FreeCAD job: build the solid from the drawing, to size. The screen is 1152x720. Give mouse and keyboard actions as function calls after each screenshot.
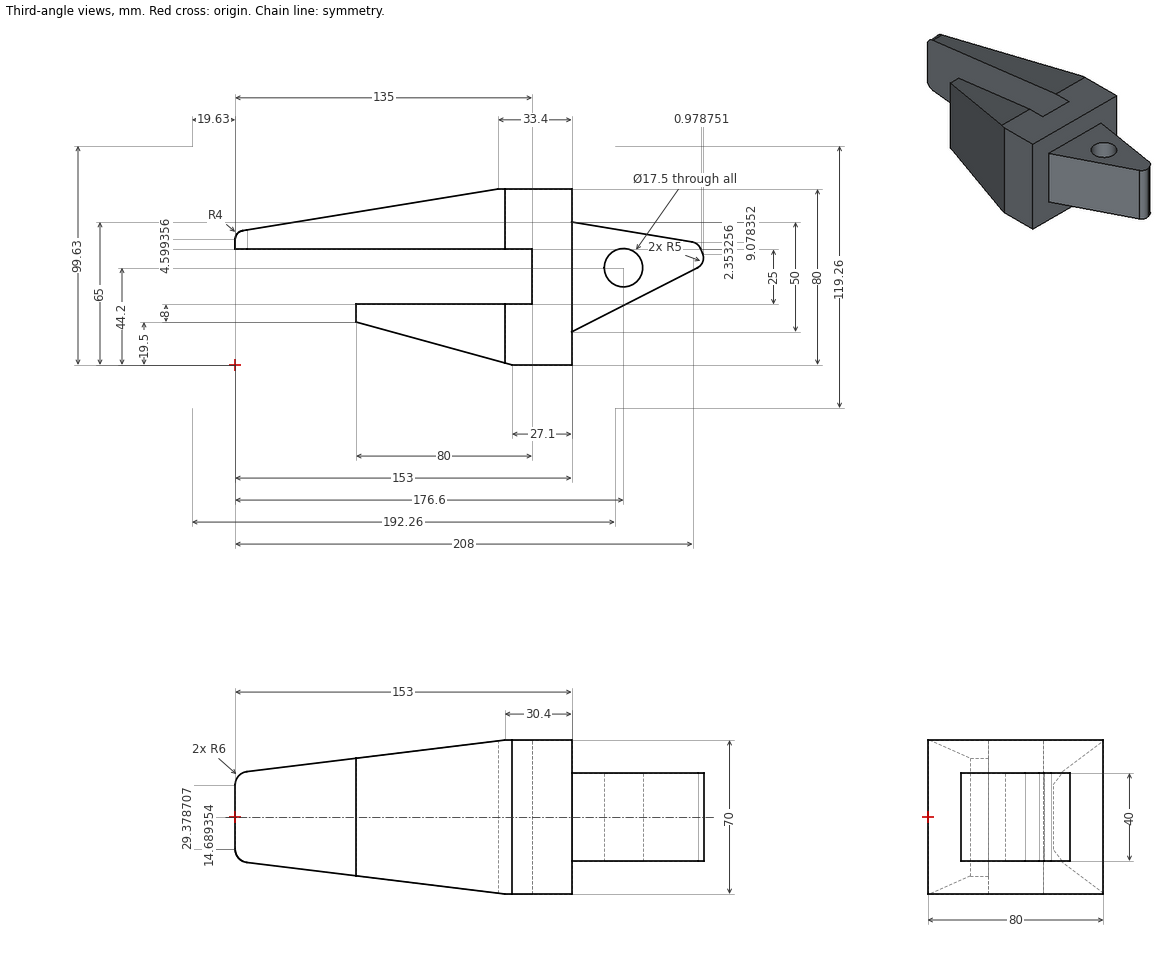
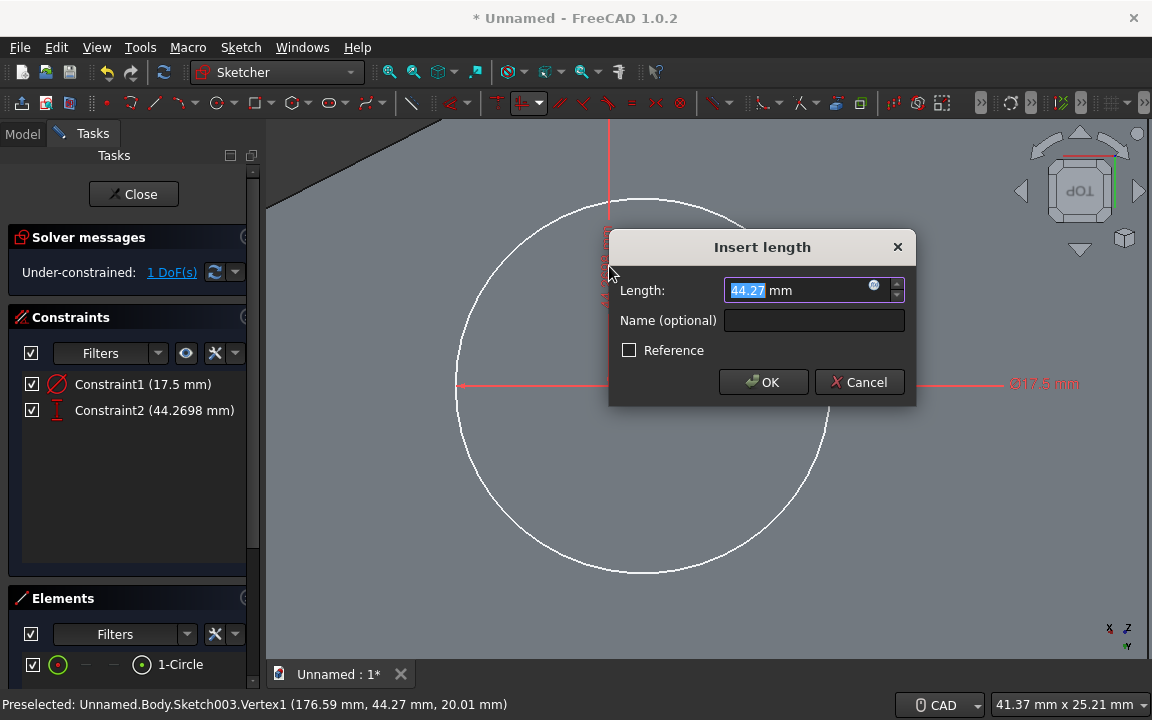
text(44.2)
key(Return)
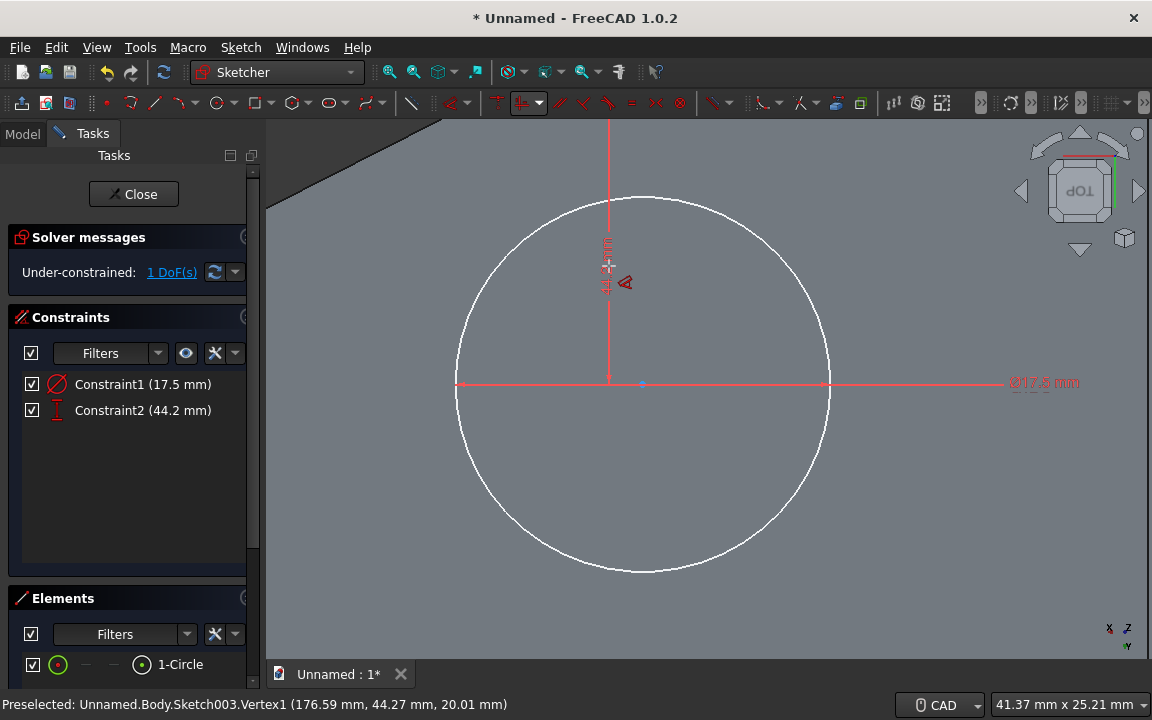
click(643, 385)
click(736, 419)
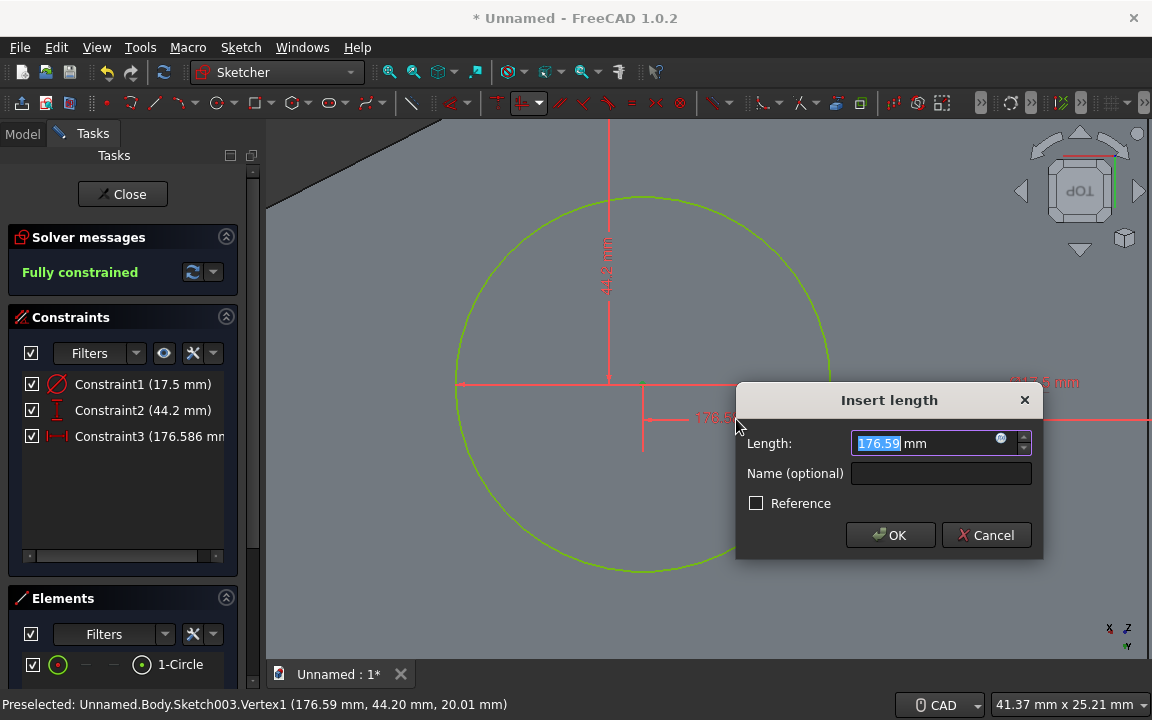
text(176.6)
key(Return)
key(Escape)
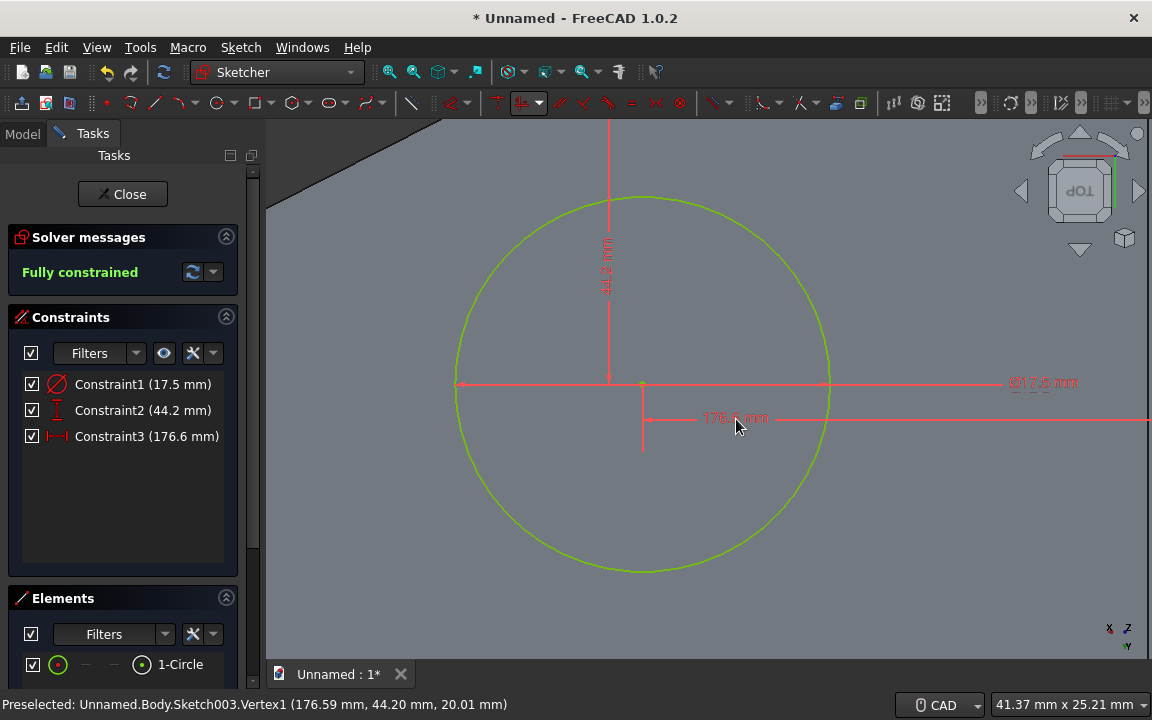
click(123, 194)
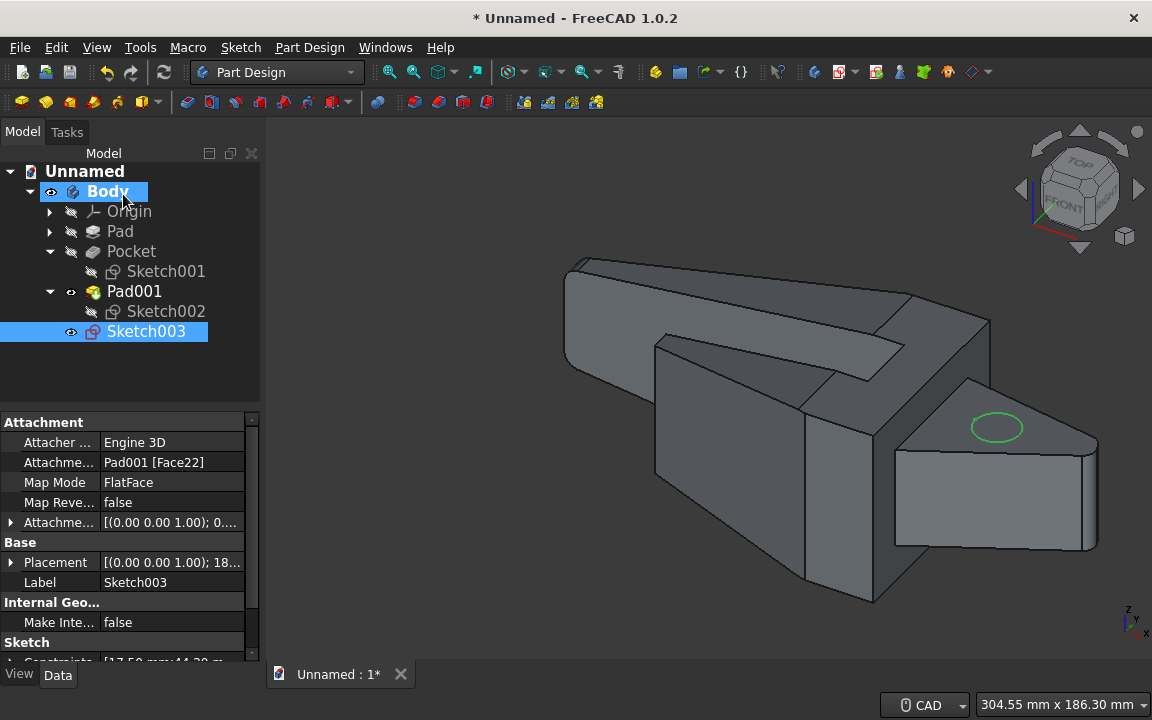
click(212, 102)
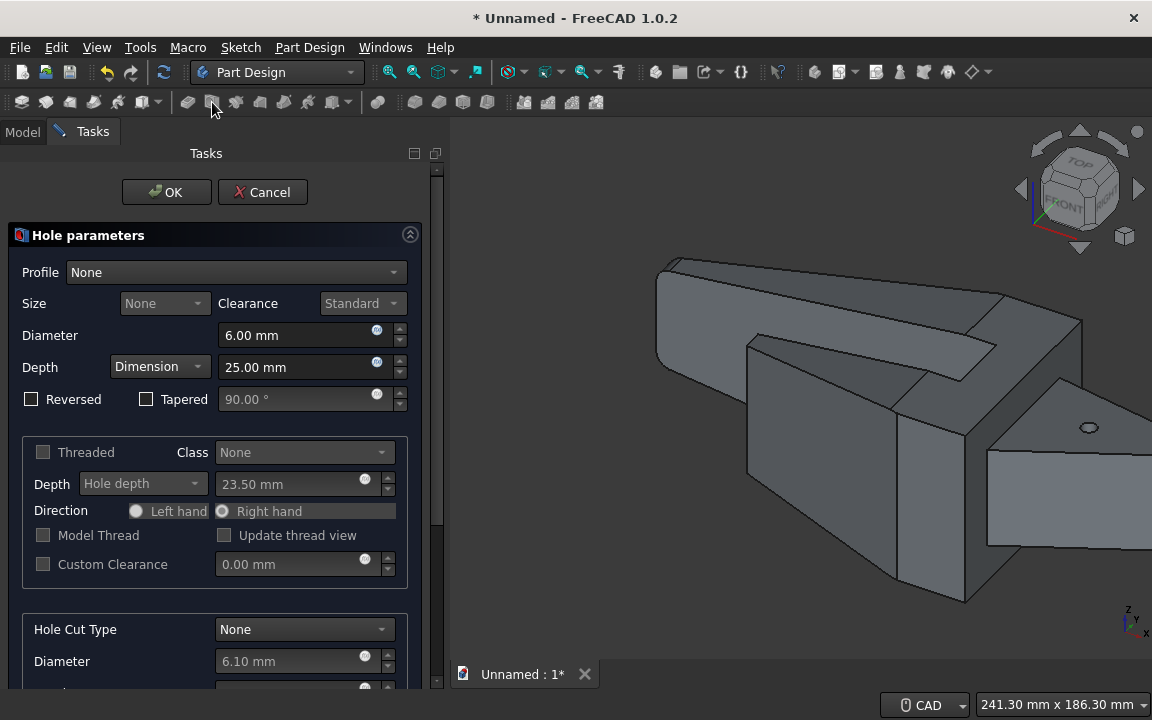
triple_click(305, 335)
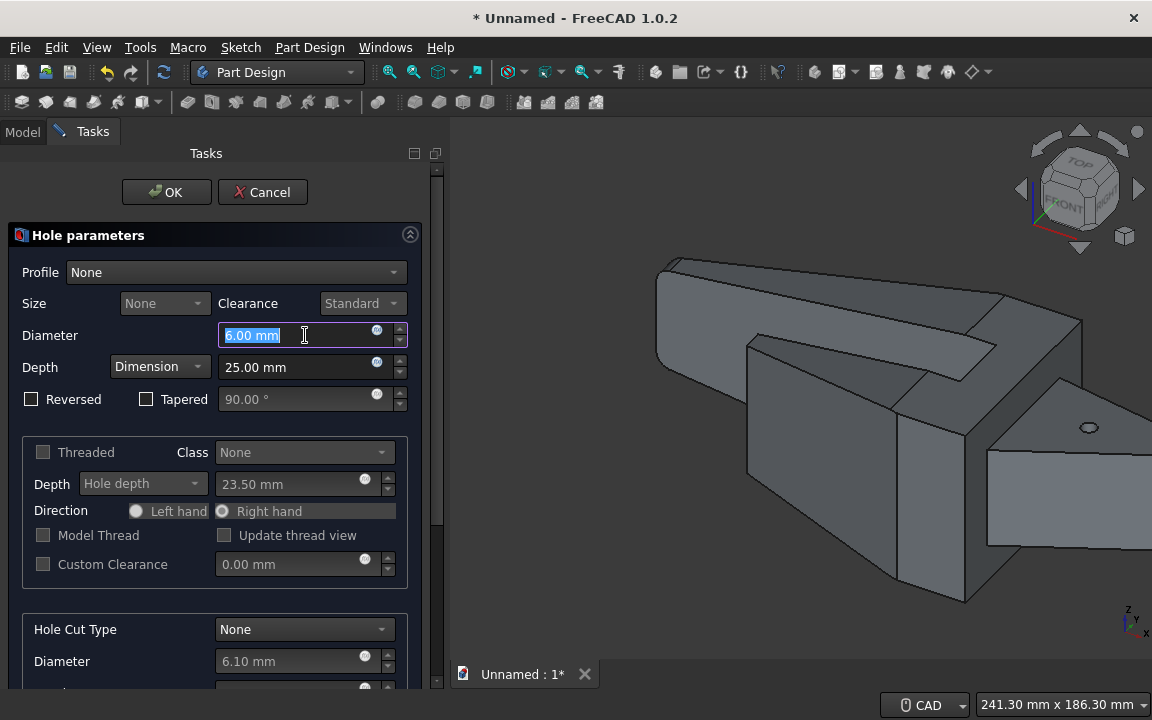
text(17.5)
key(Tab)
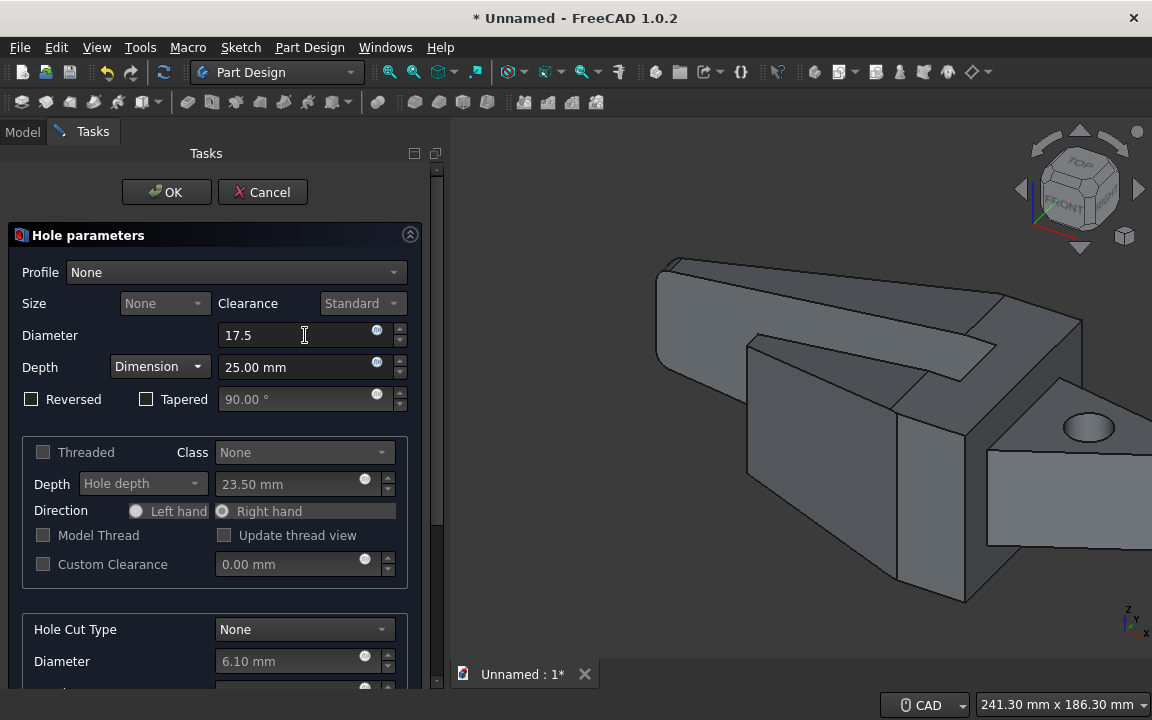
click(161, 366)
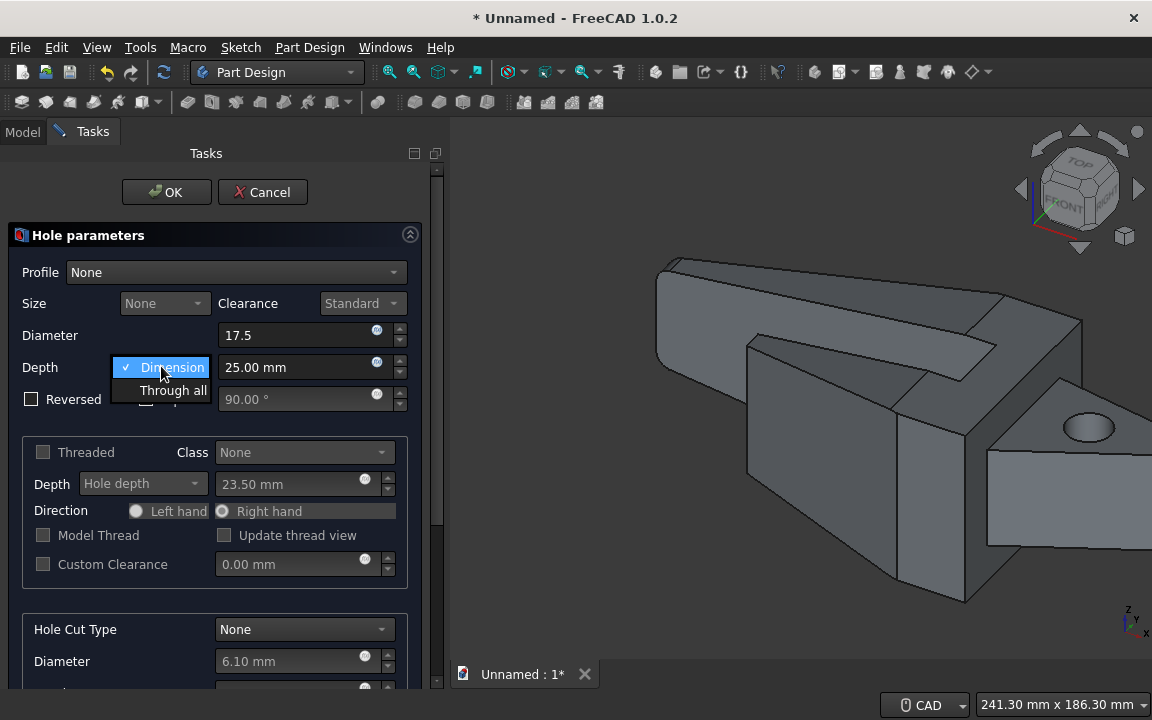
click(160, 390)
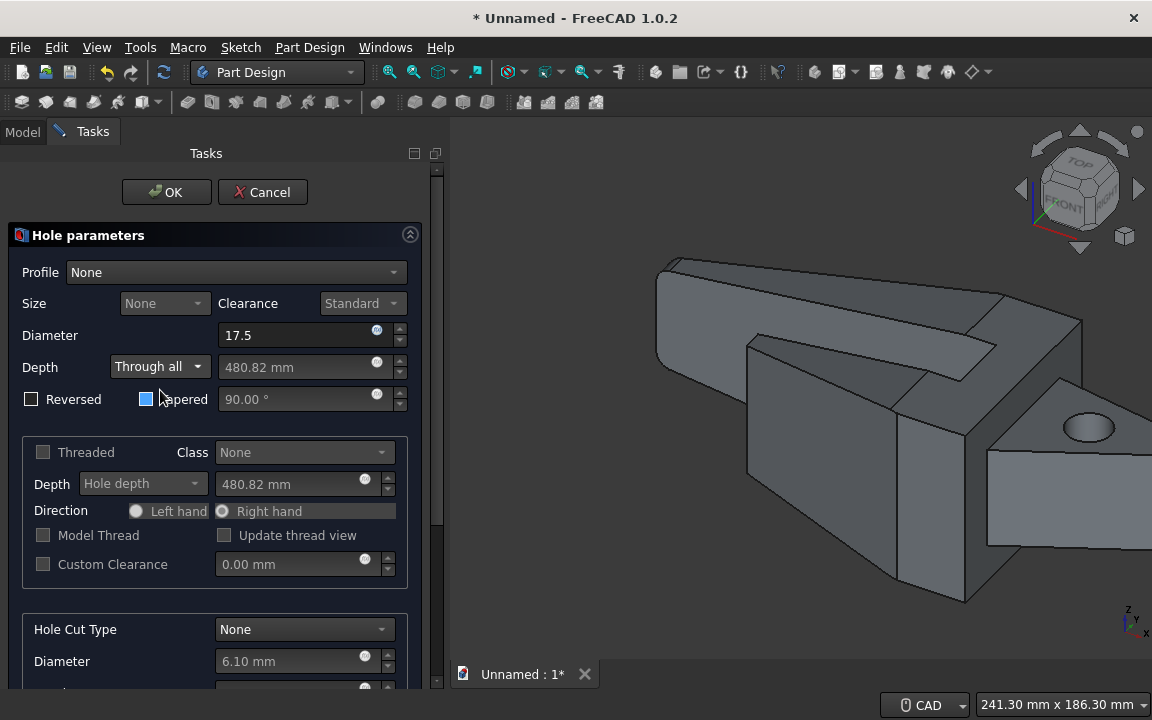
click(167, 192)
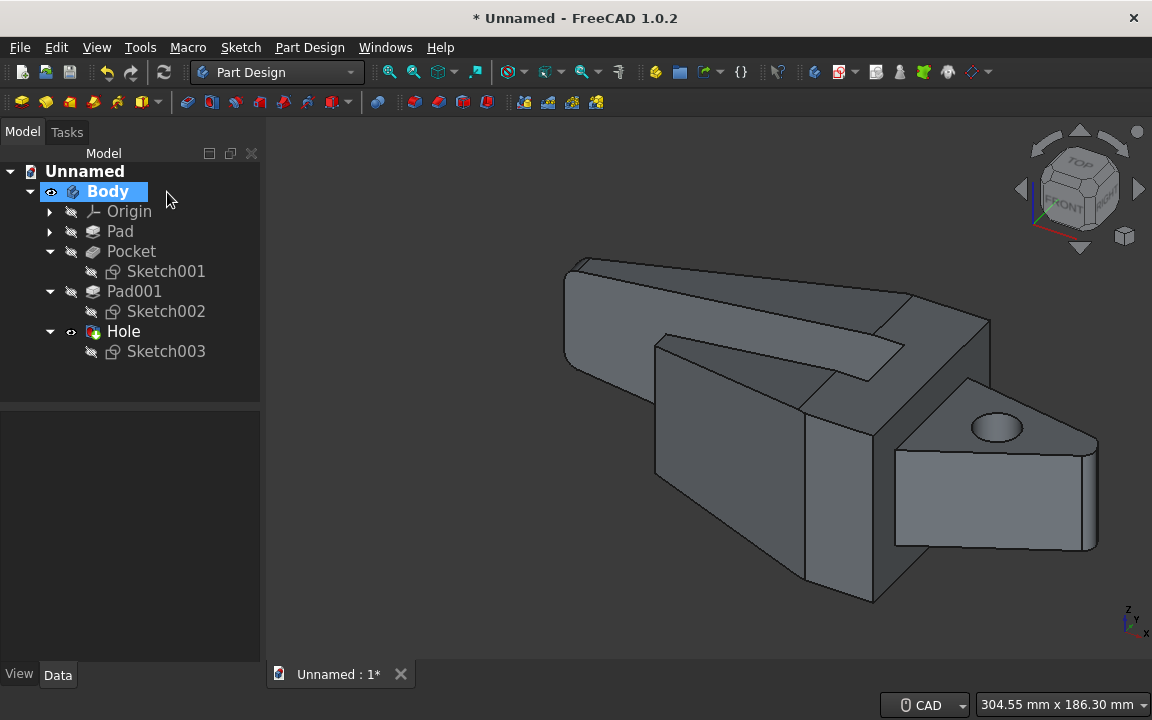
key(0)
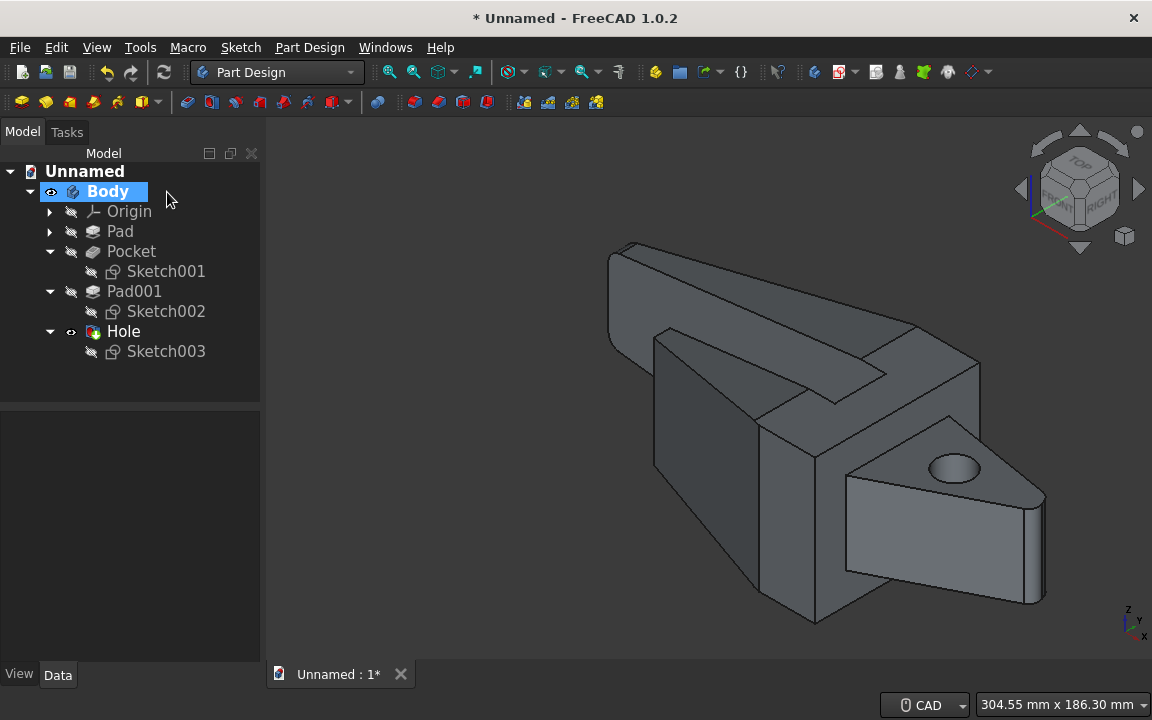
click(390, 72)